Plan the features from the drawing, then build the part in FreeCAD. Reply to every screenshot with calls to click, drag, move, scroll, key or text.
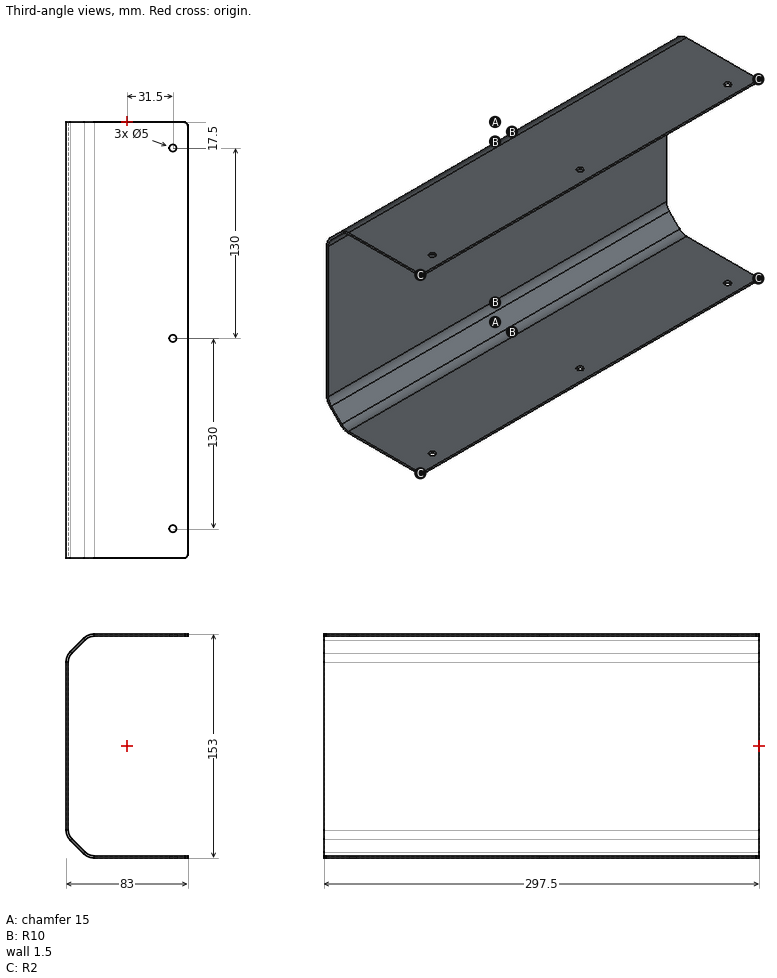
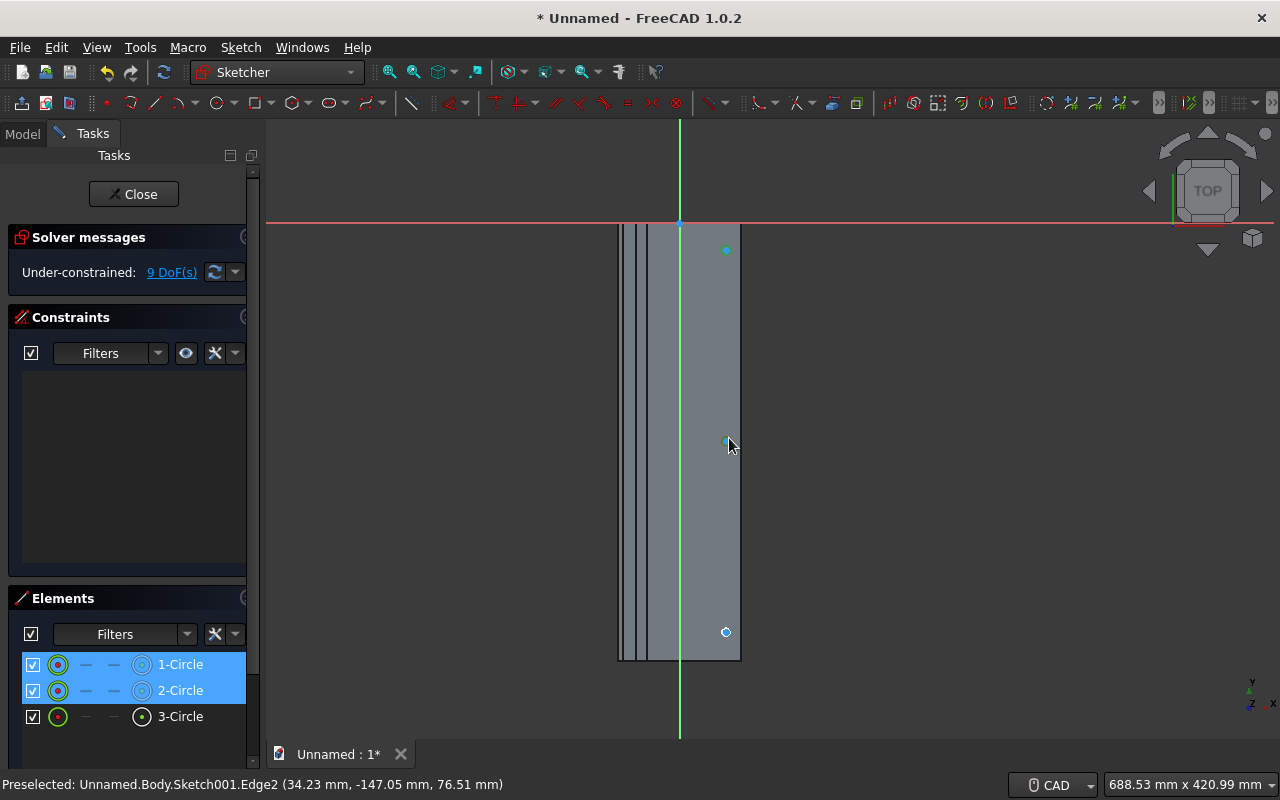
scroll(729, 630, up, 7)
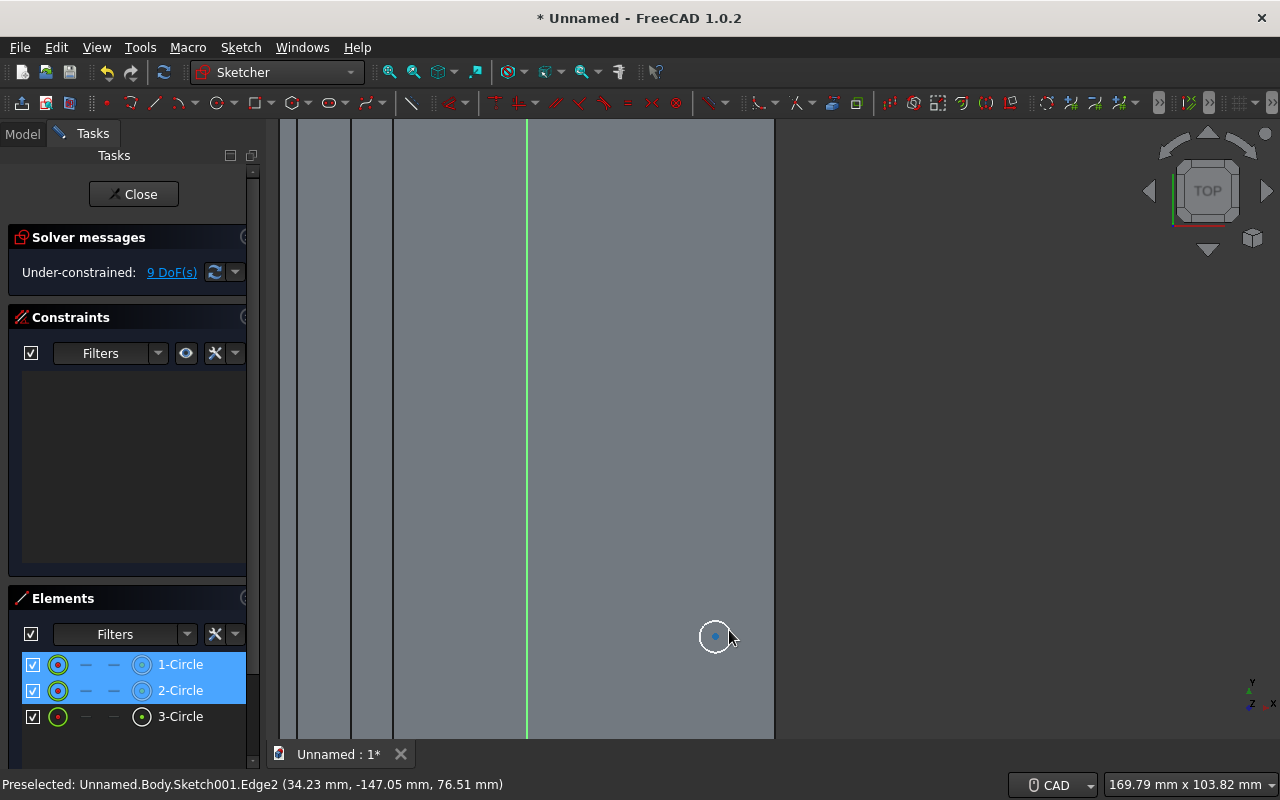
click(727, 626)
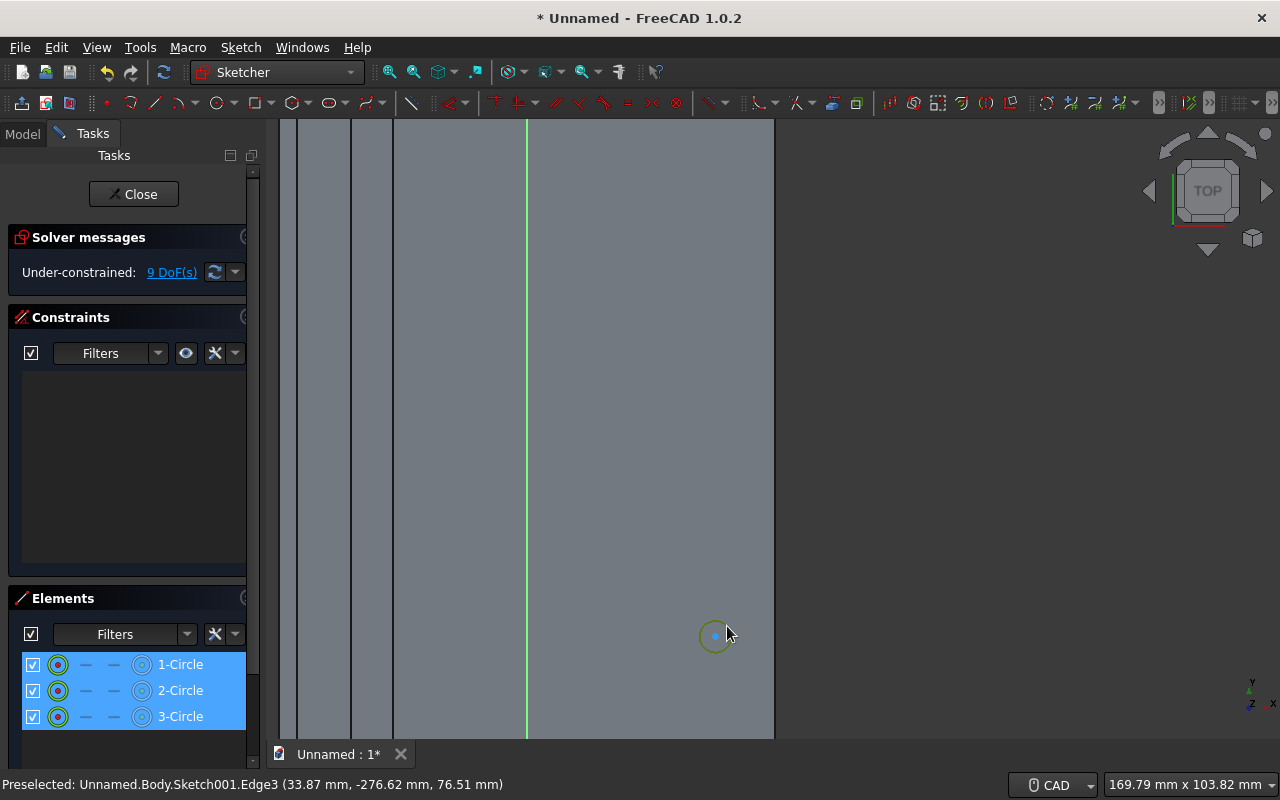
key(e)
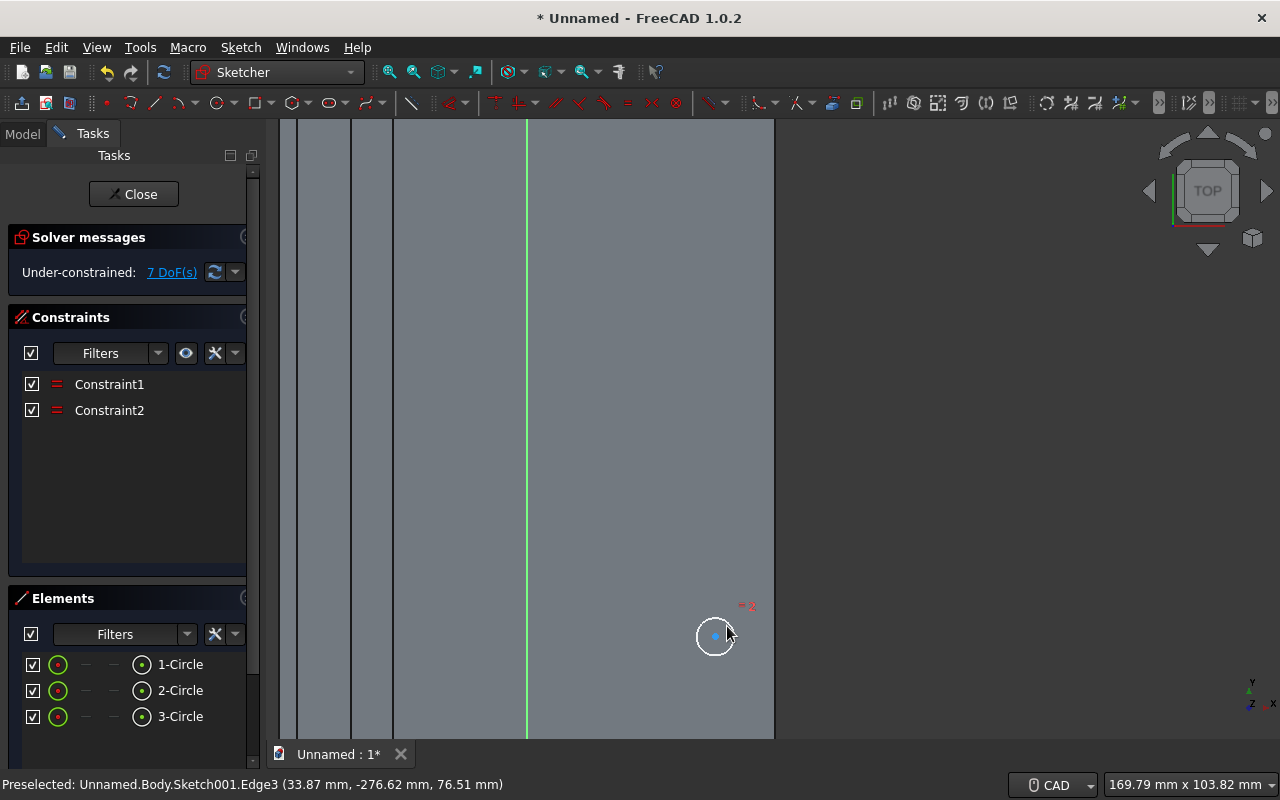
scroll(729, 631, down, 7)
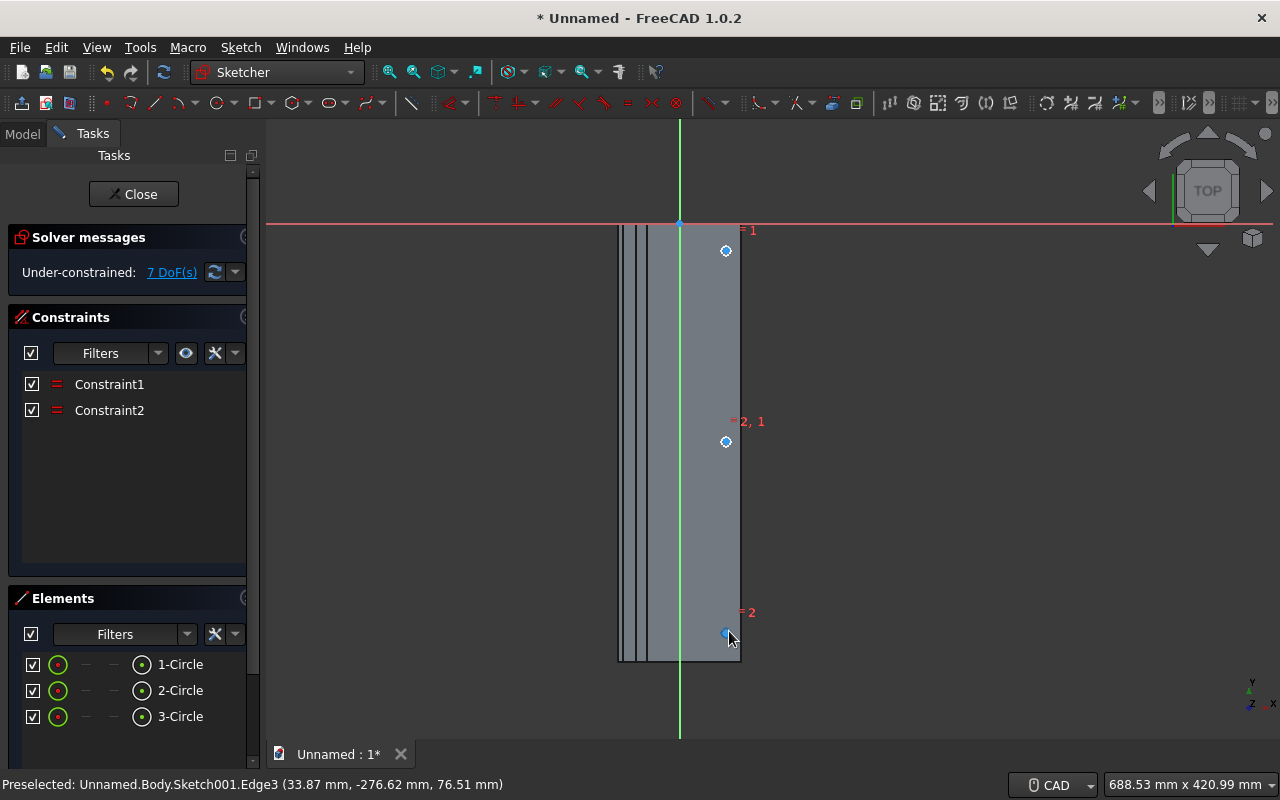
click(726, 251)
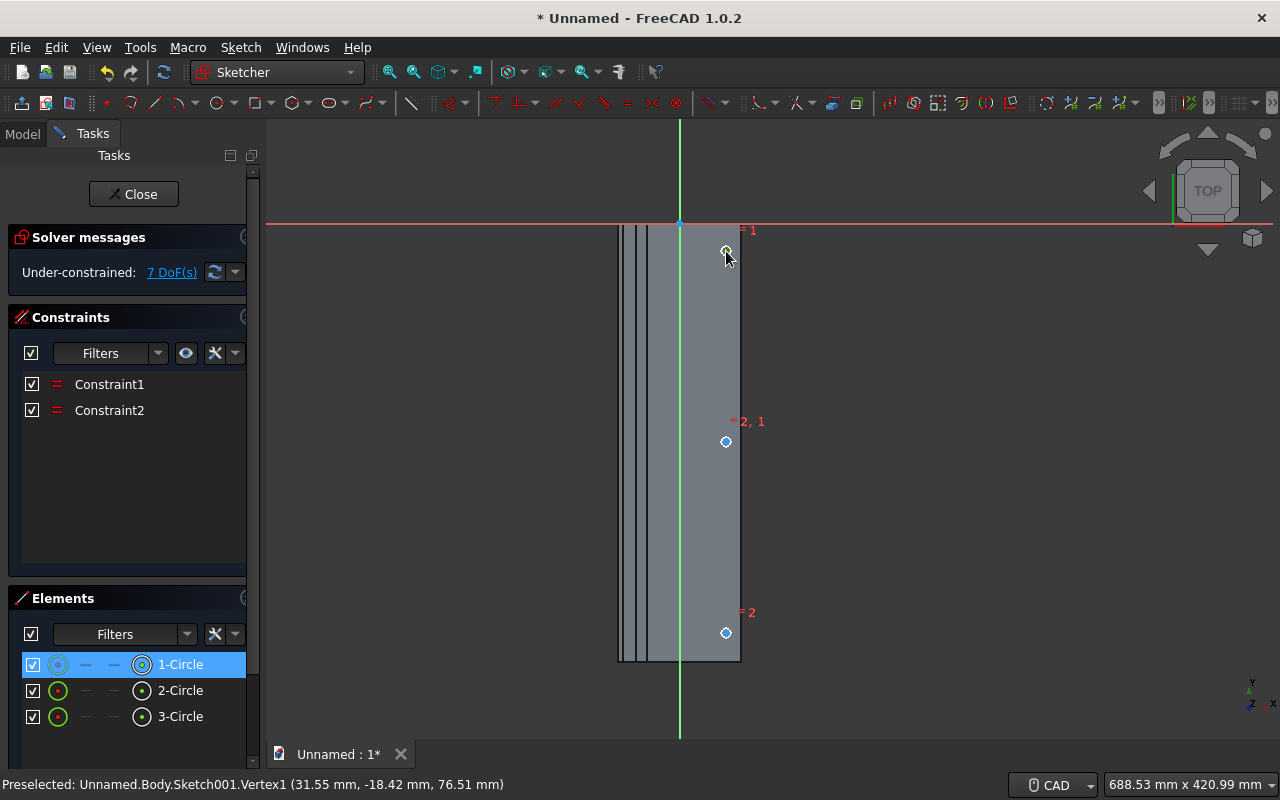
click(726, 442)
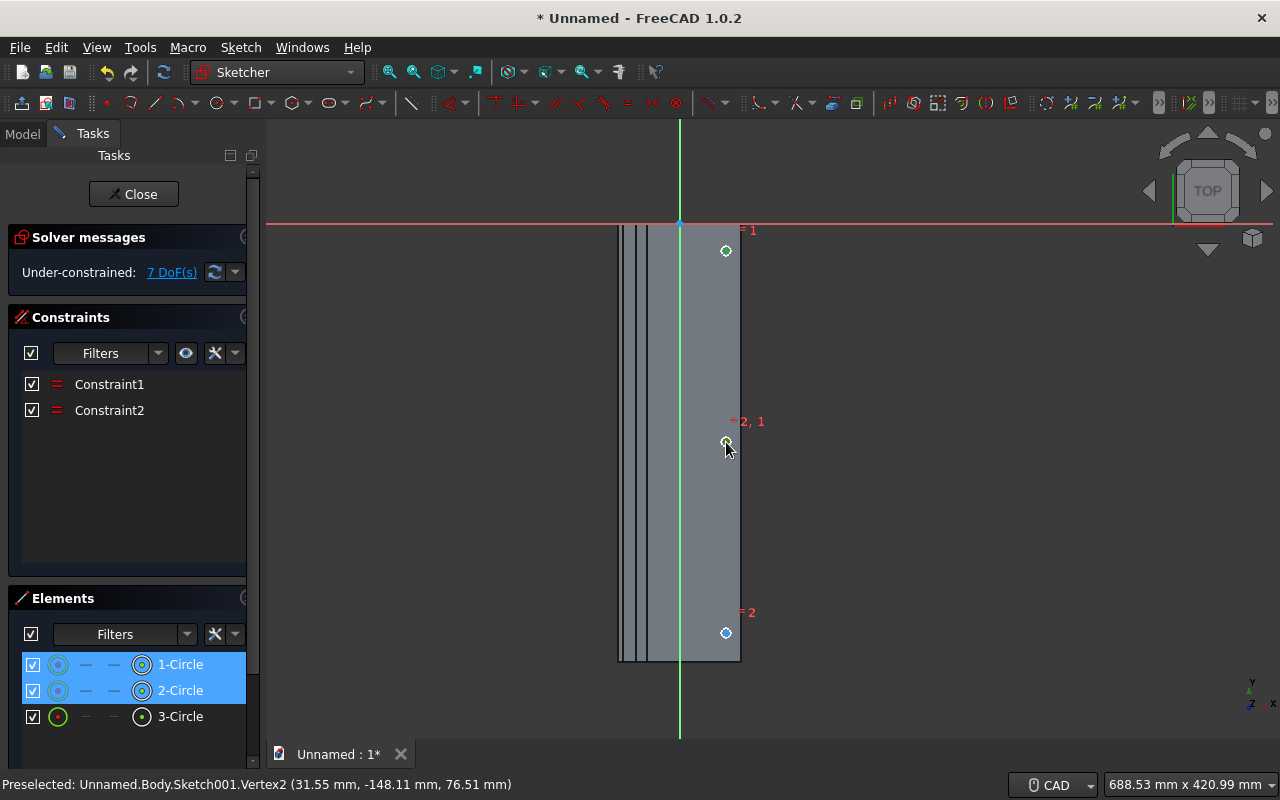
key(v)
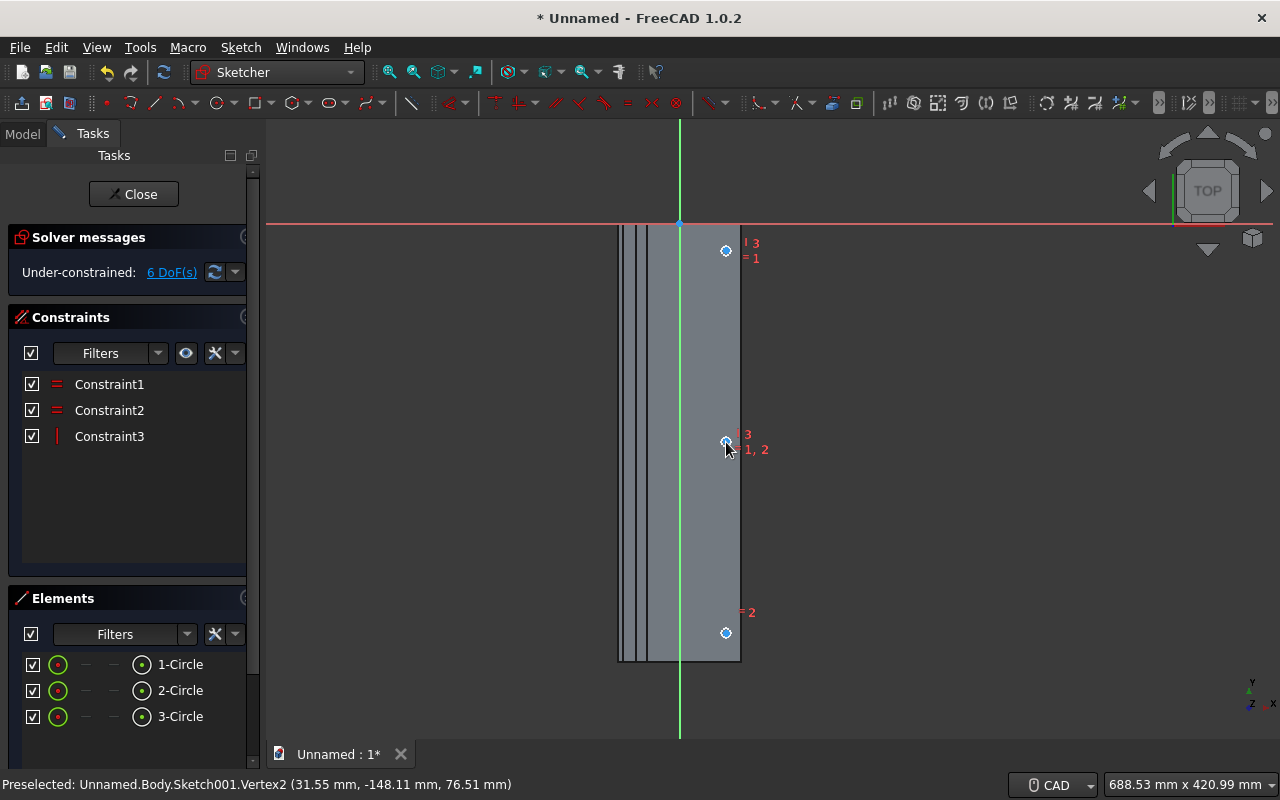
click(726, 442)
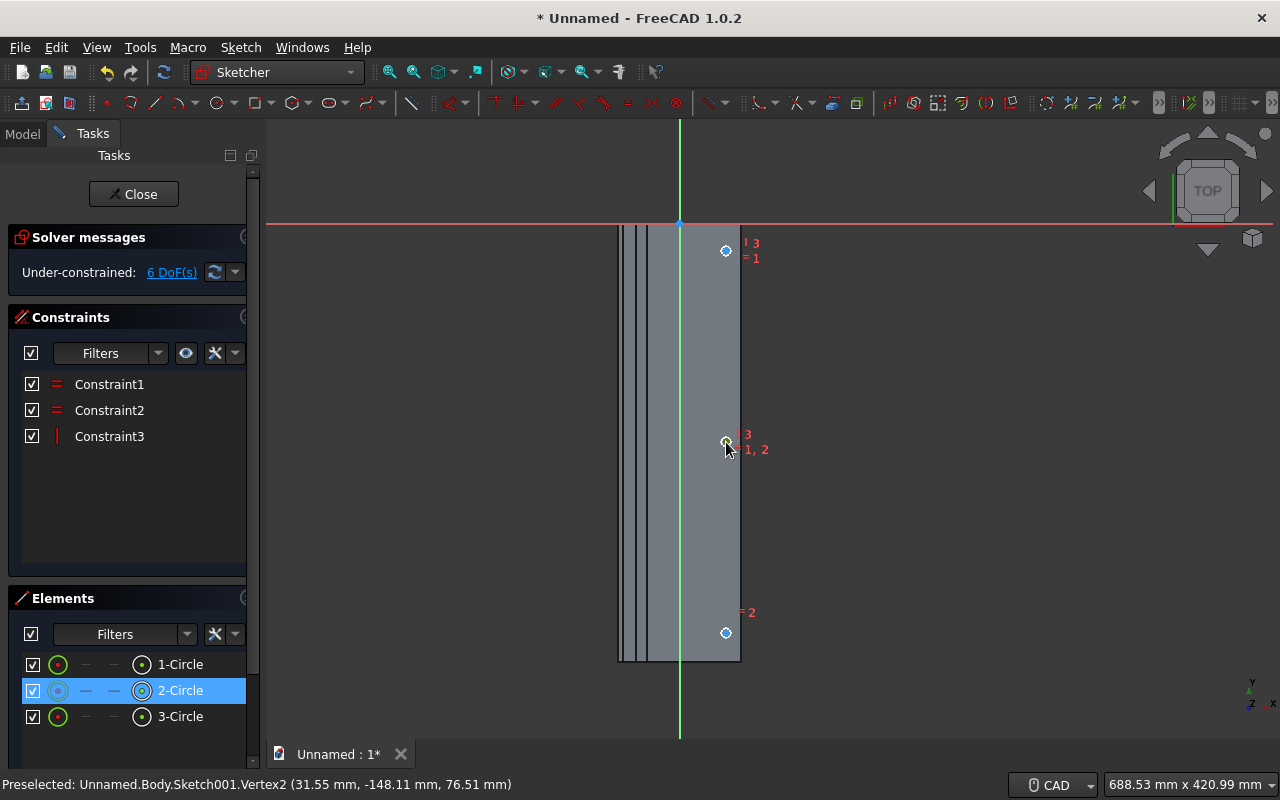
click(726, 633)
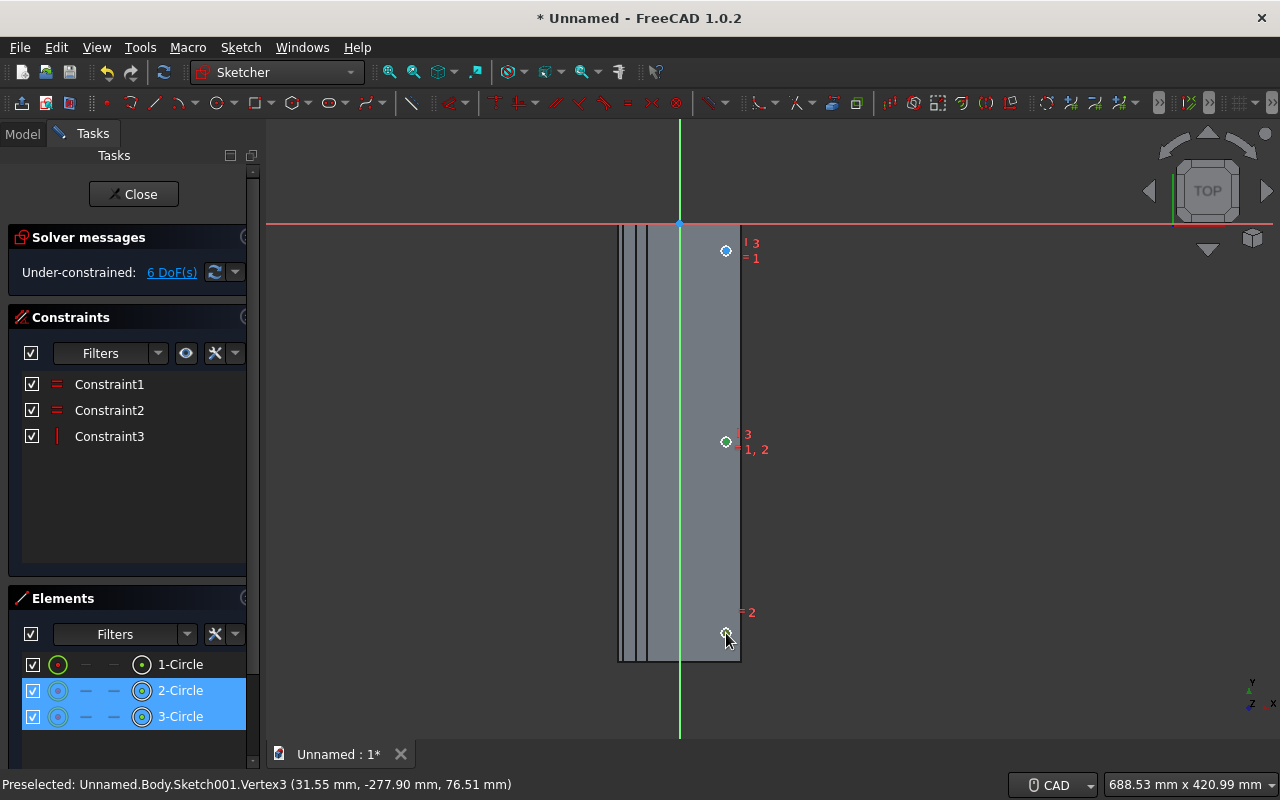
key(v)